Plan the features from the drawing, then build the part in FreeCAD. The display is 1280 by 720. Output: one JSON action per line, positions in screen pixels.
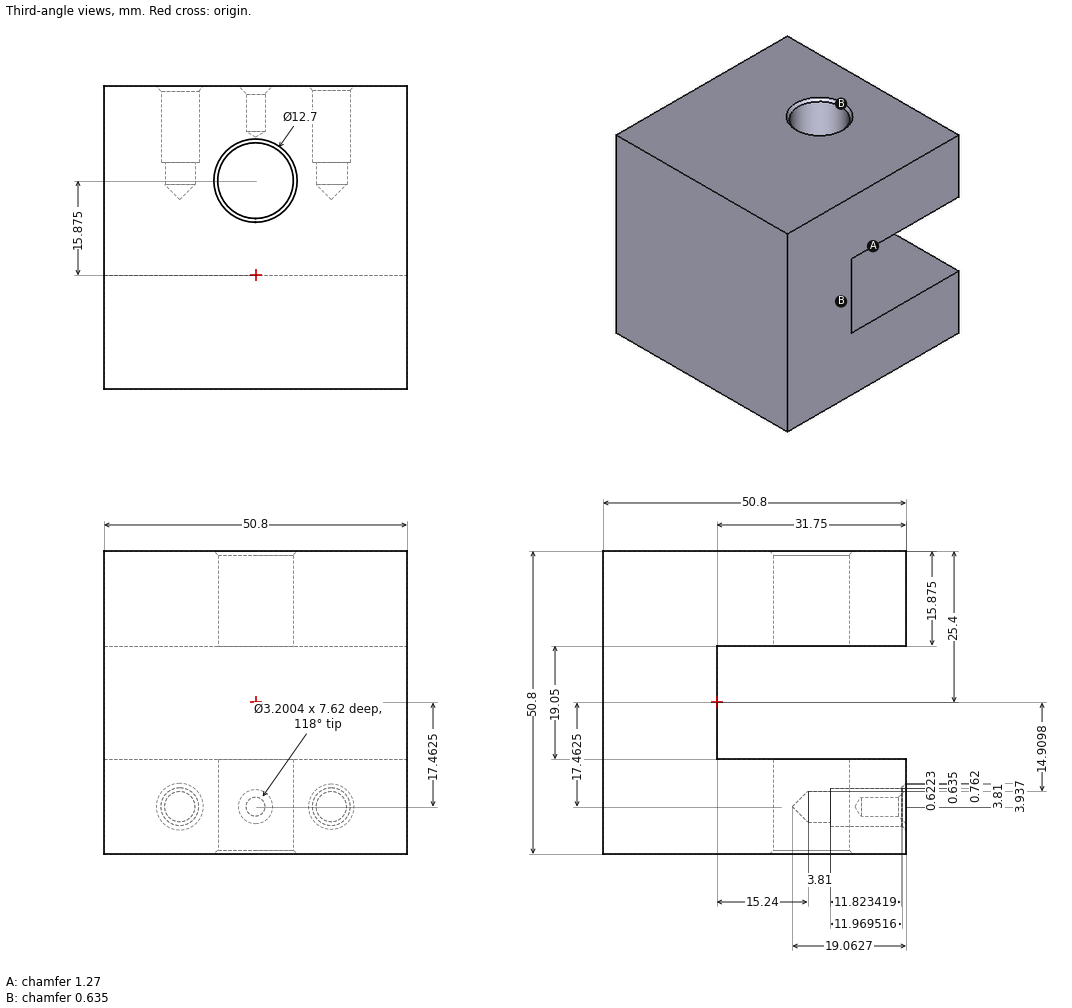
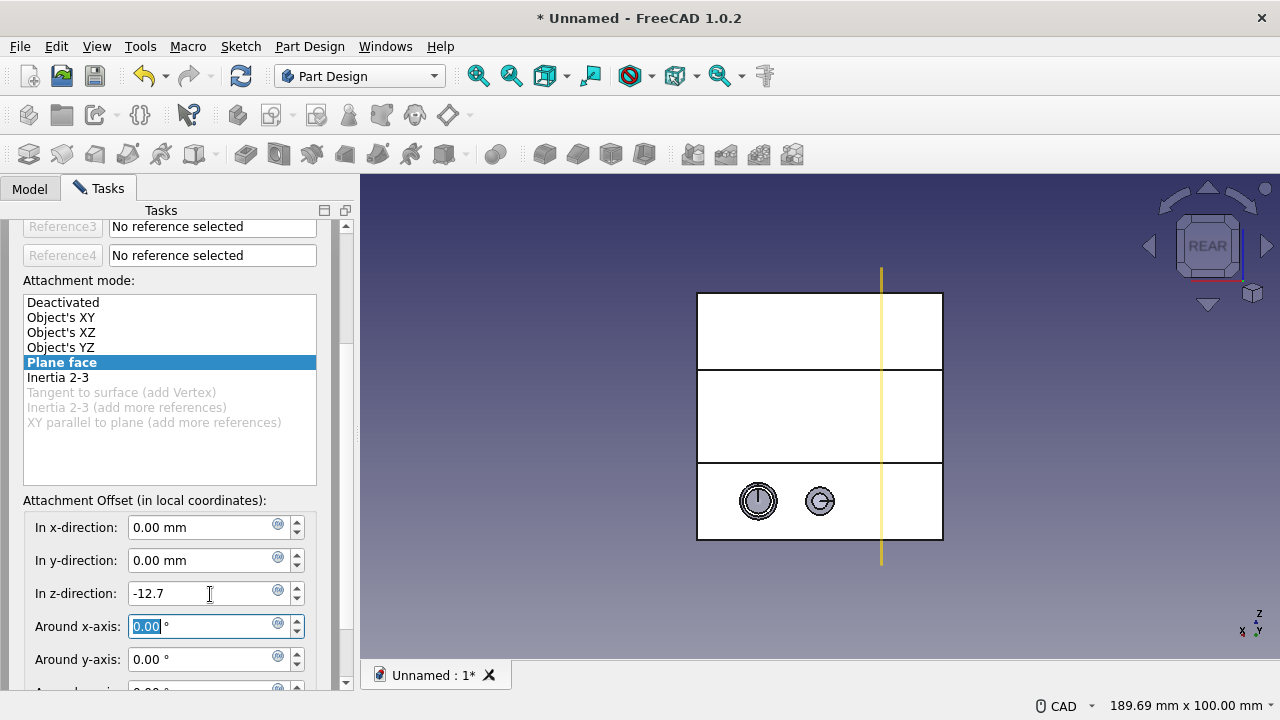
{"action": "scroll", "coordinate": [346, 455], "scroll_direction": "up", "scroll_amount": 4}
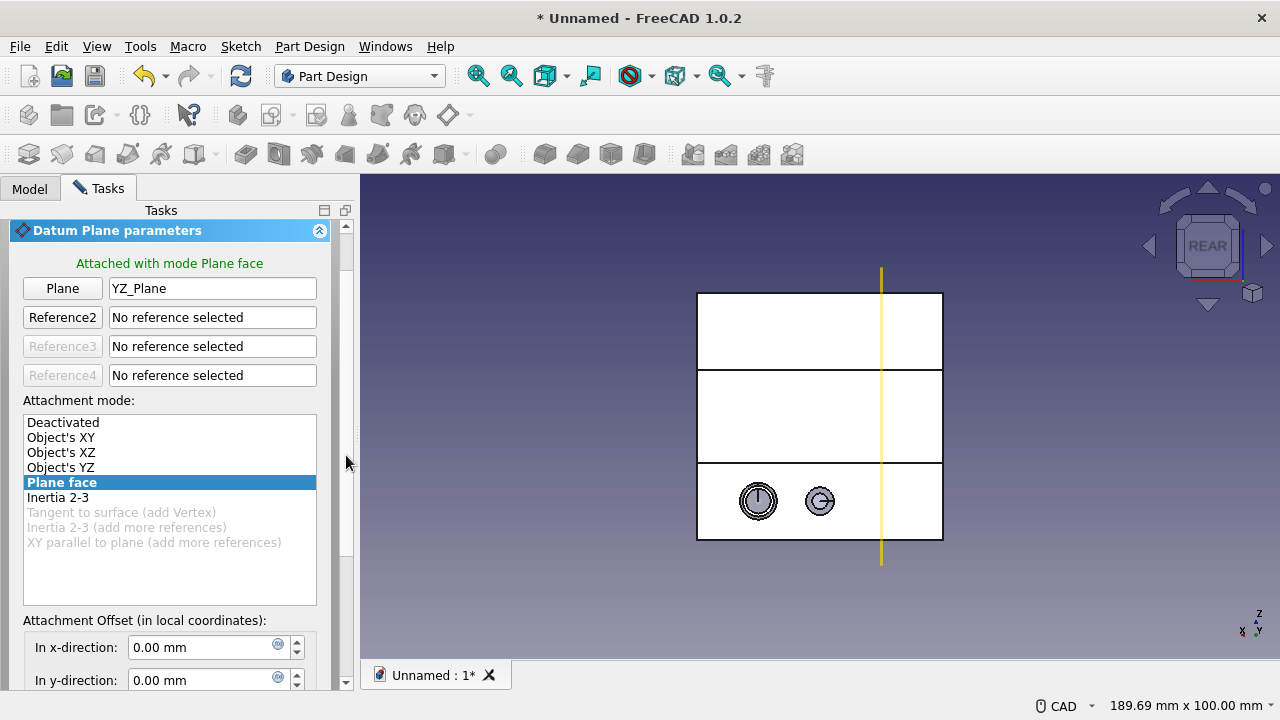
{"action": "left_click", "coordinate": [127, 249]}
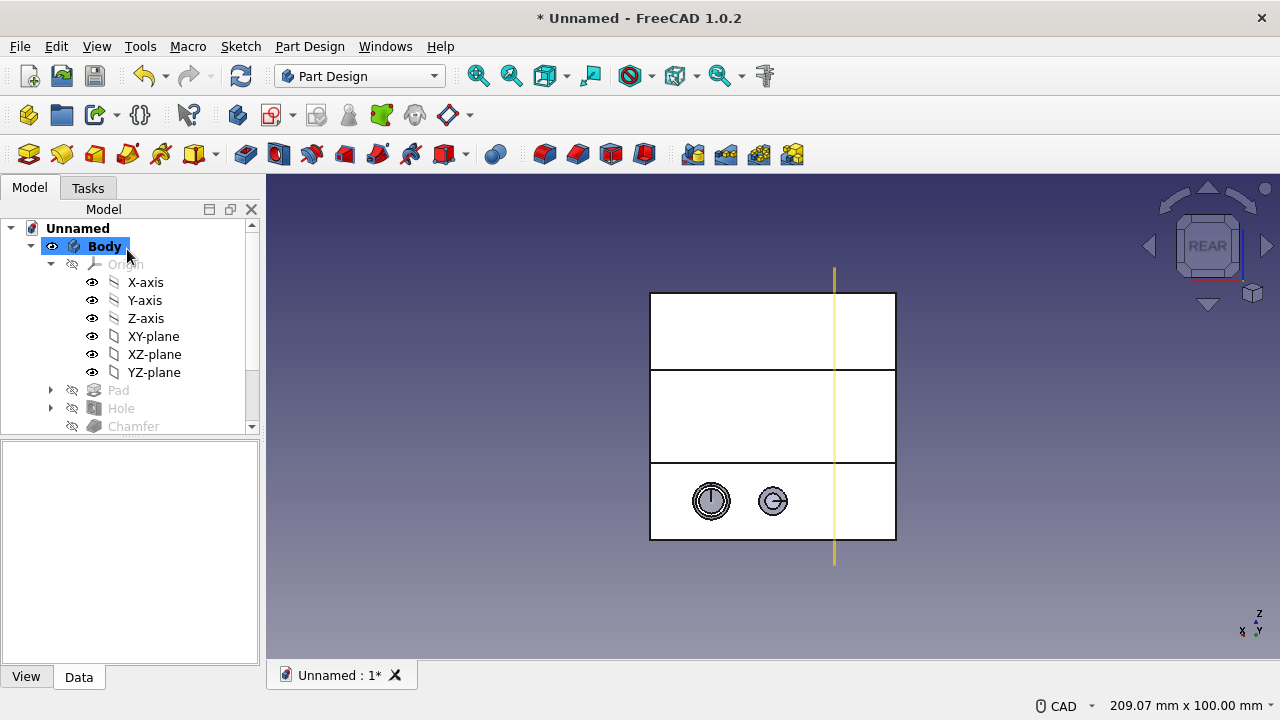
{"action": "scroll", "coordinate": [101, 332], "scroll_direction": "down", "scroll_amount": 3}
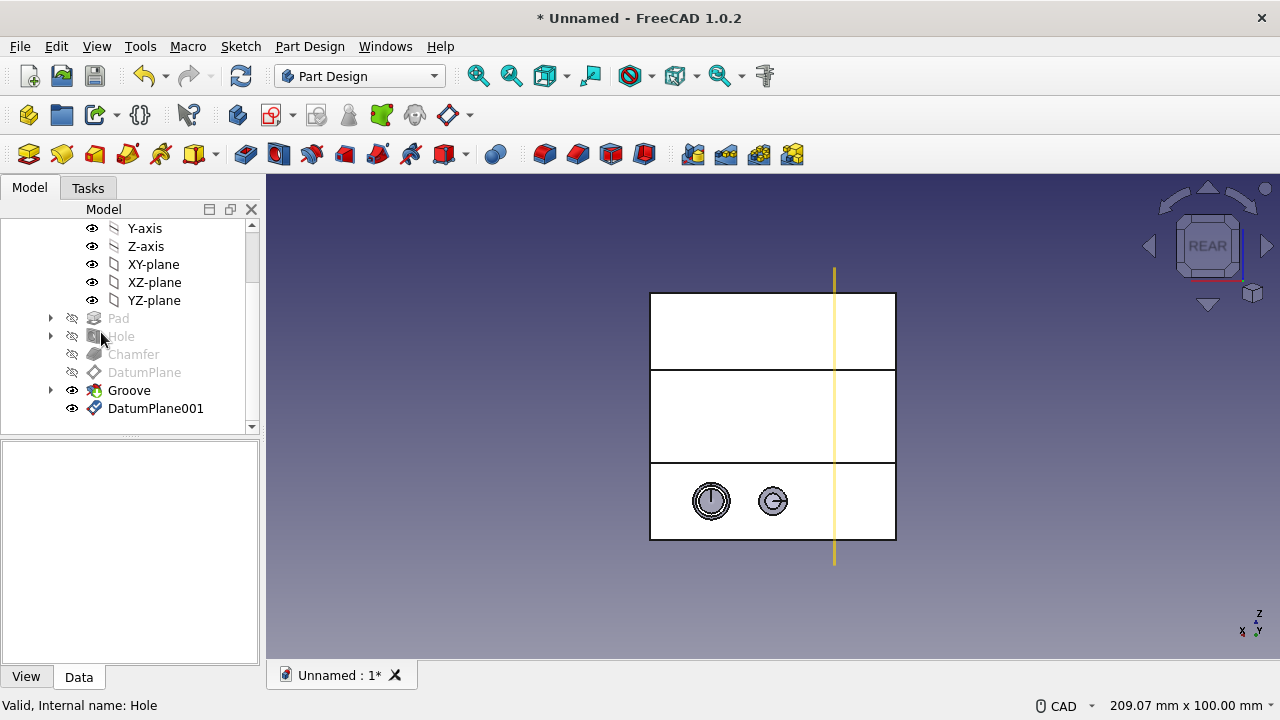
{"action": "left_click", "coordinate": [117, 408]}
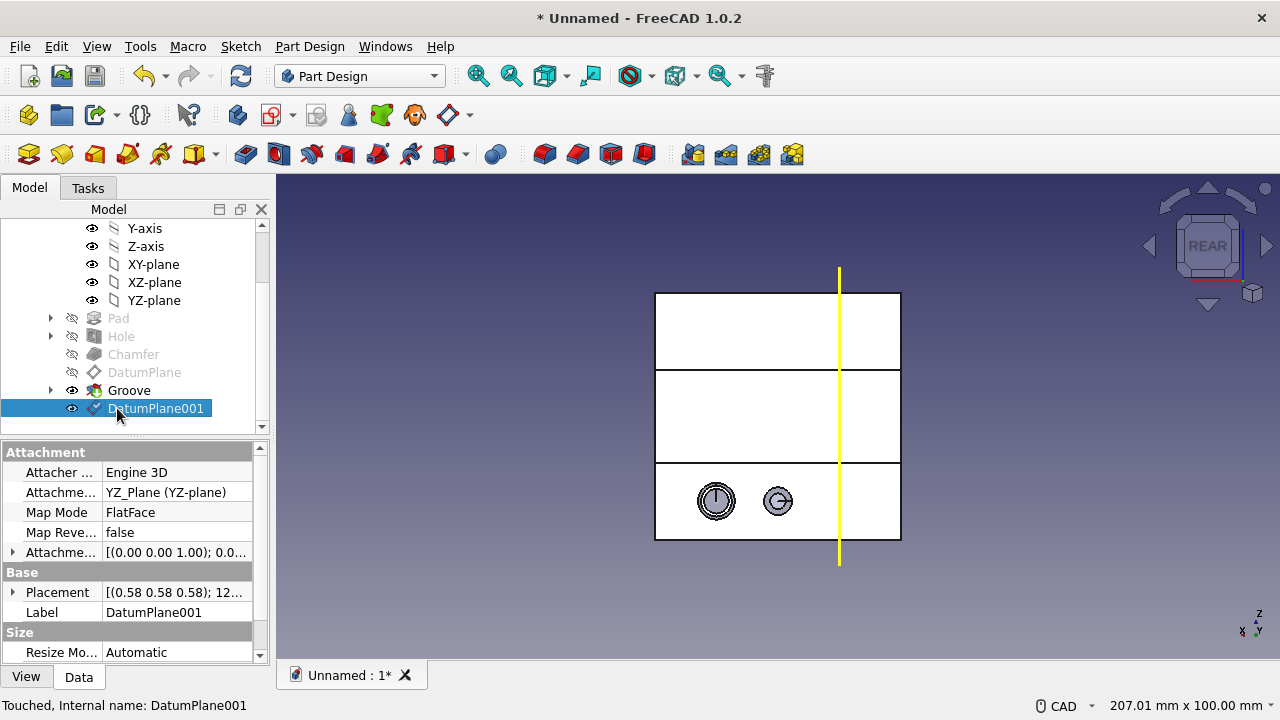
{"action": "left_click", "coordinate": [270, 116]}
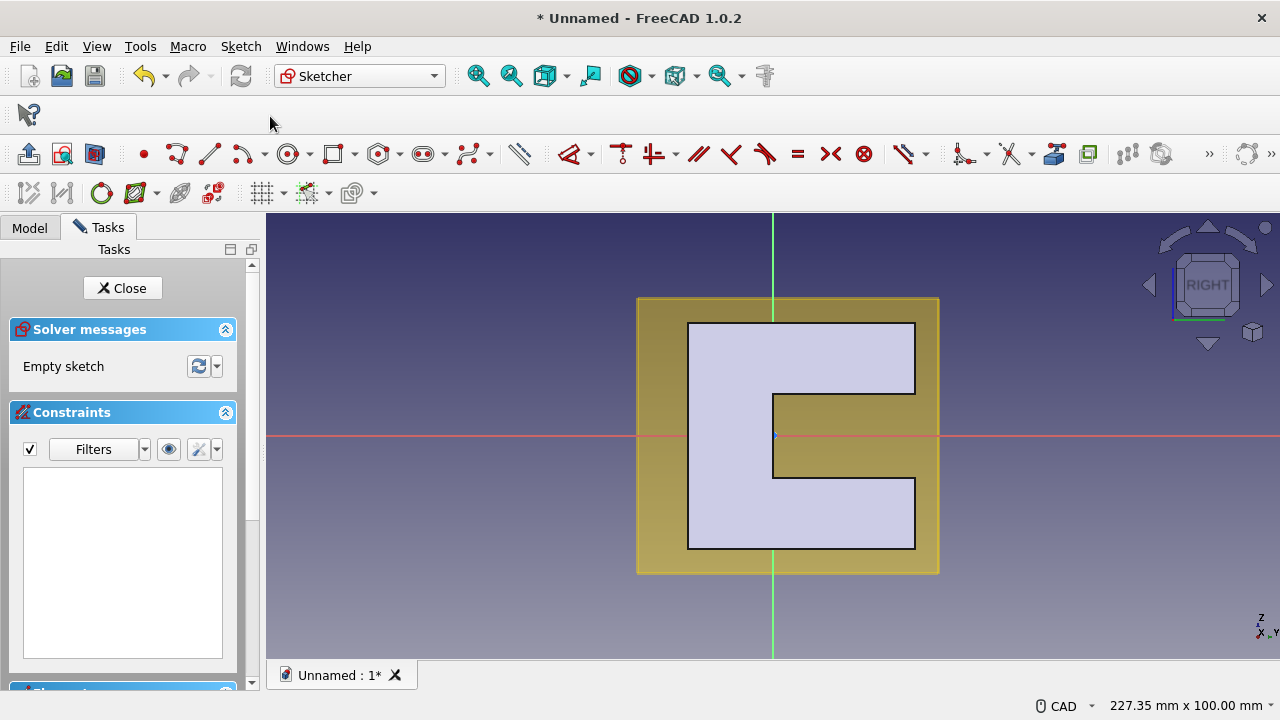
{"action": "left_click", "coordinate": [95, 154]}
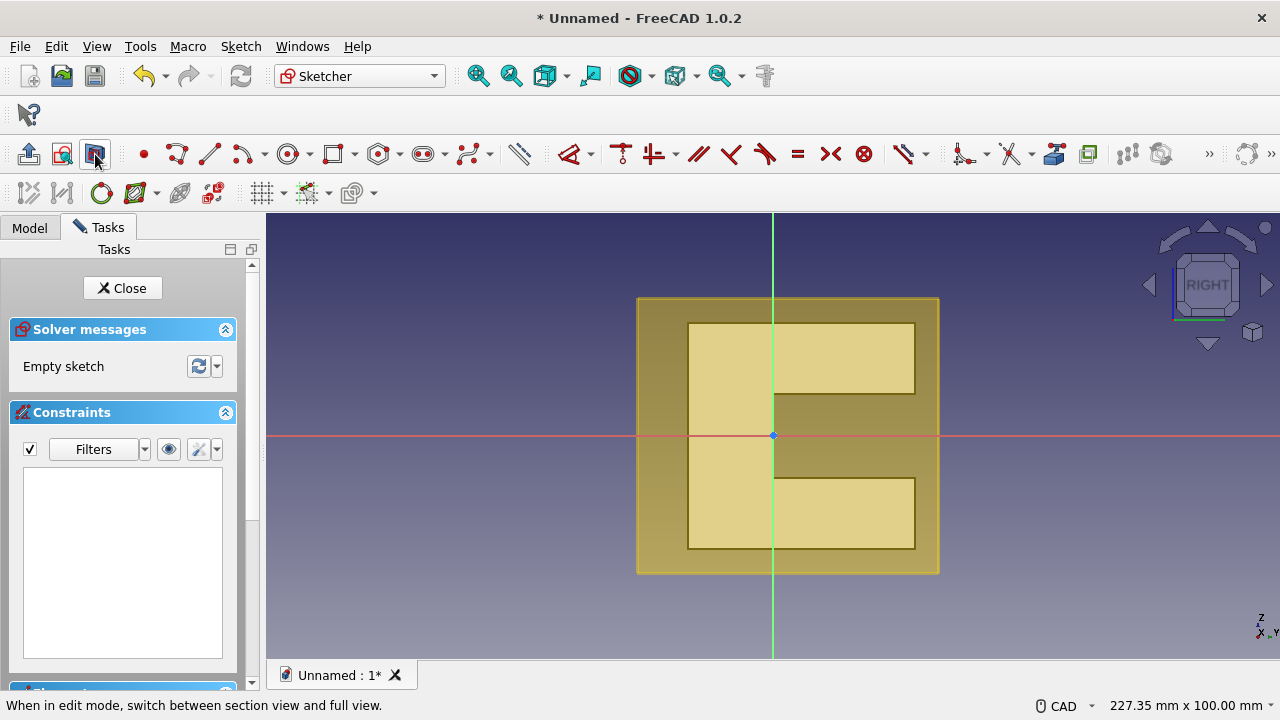
{"action": "scroll", "coordinate": [904, 492], "scroll_direction": "up", "scroll_amount": 6}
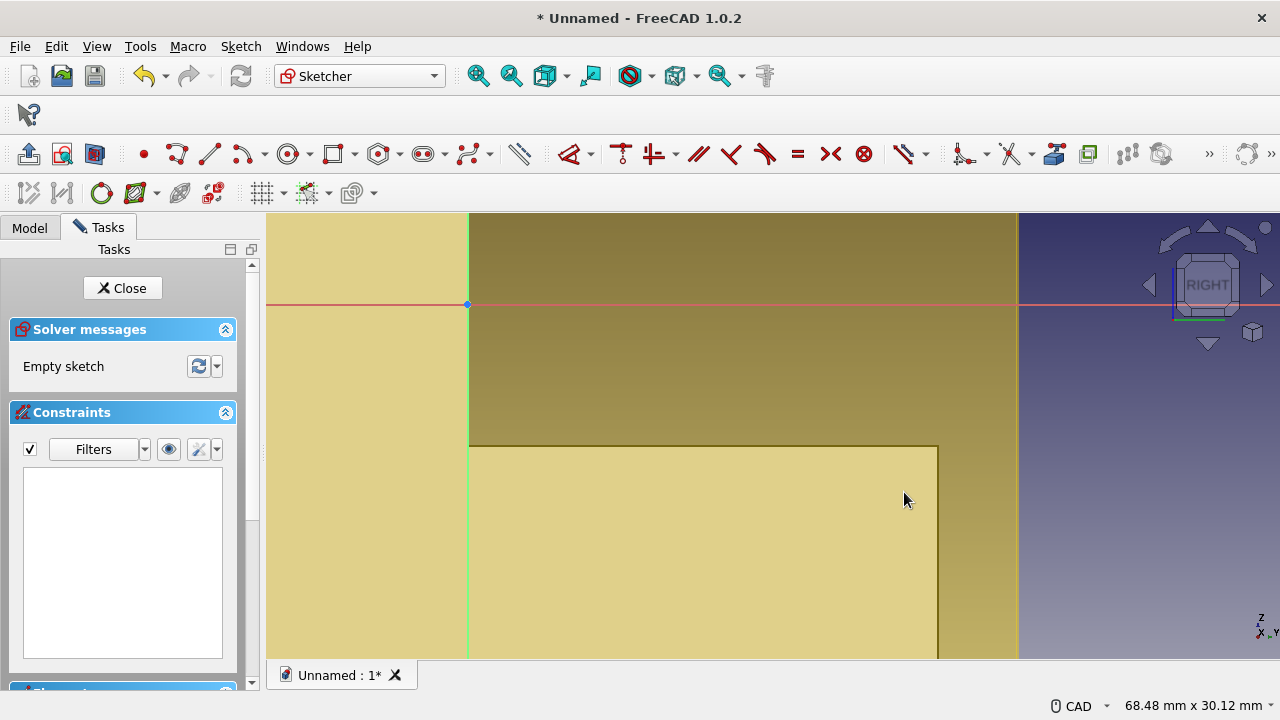
{"action": "left_click", "coordinate": [177, 154]}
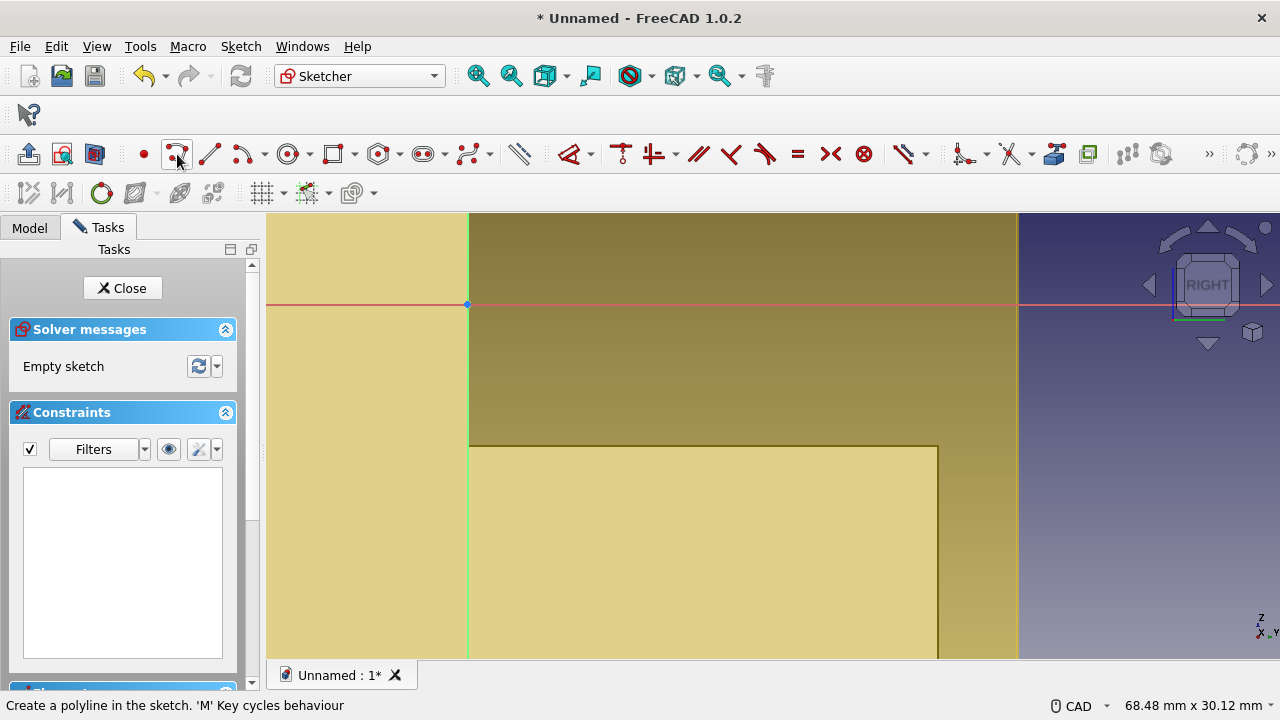
{"action": "left_click", "coordinate": [693, 525]}
{"action": "left_click", "coordinate": [655, 563]}
{"action": "left_click", "coordinate": [938, 563]}
{"action": "left_click", "coordinate": [938, 505]}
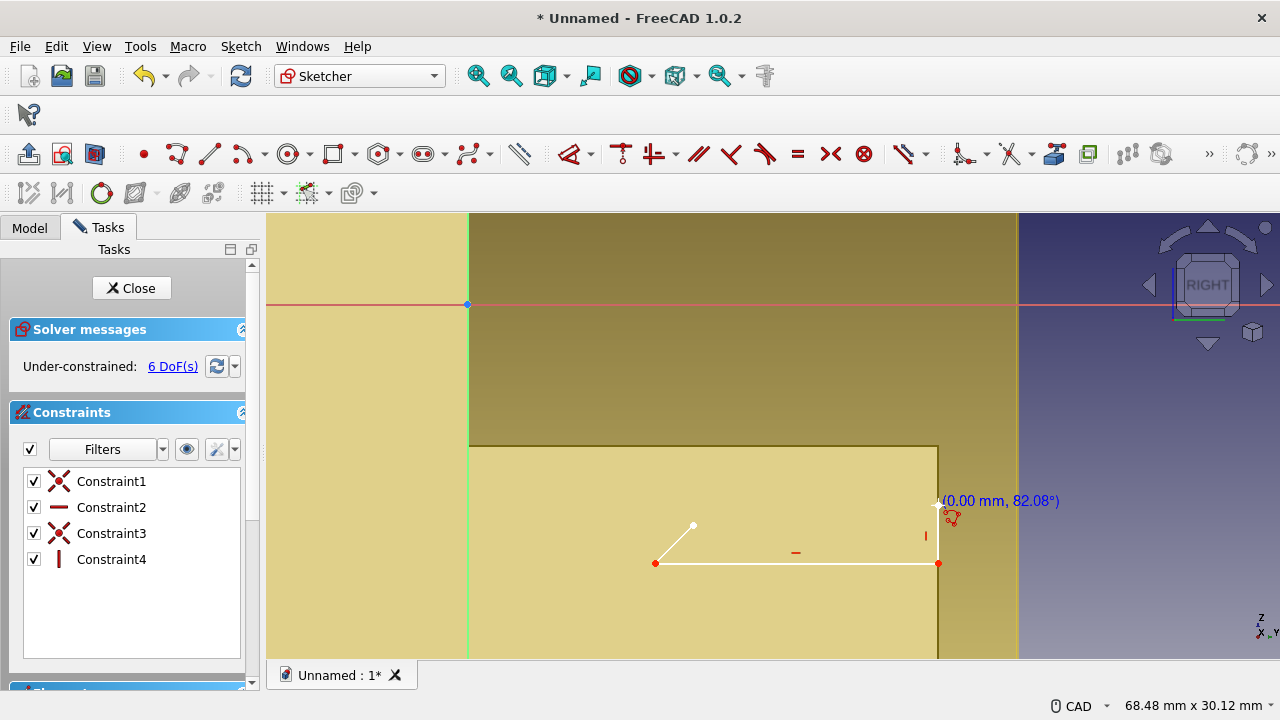
{"action": "scroll", "coordinate": [925, 516], "scroll_direction": "up", "scroll_amount": 2}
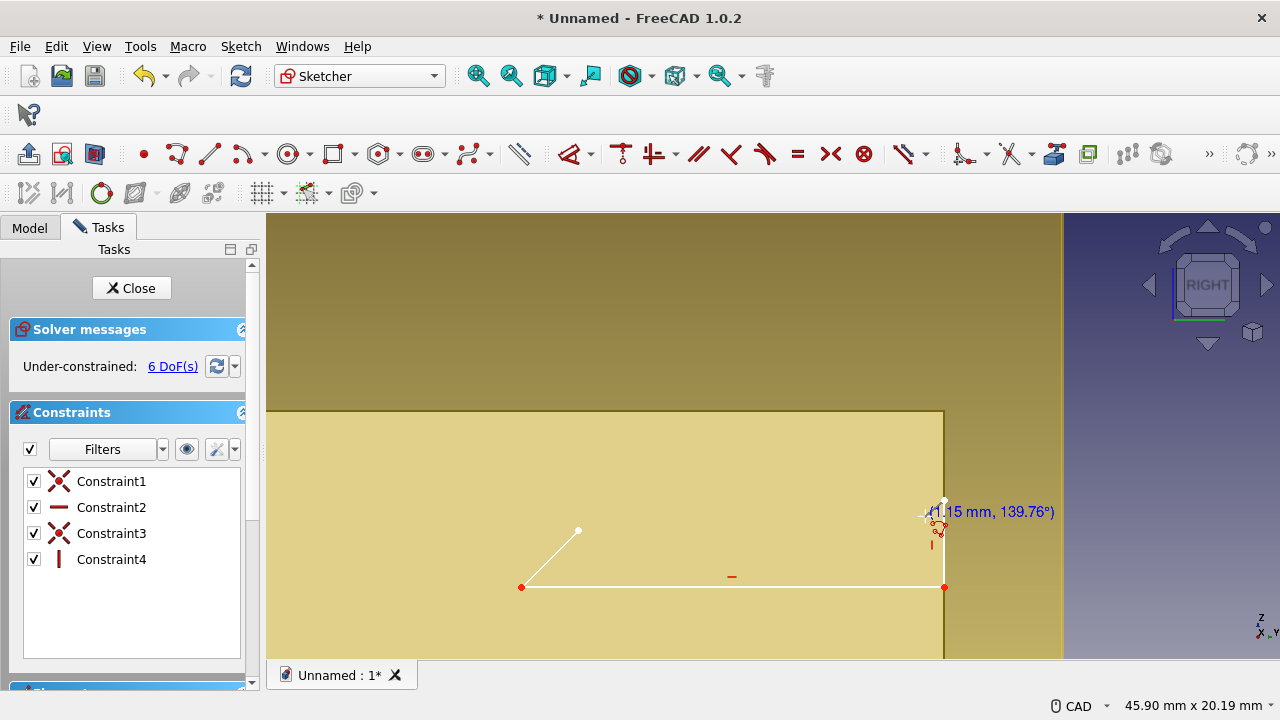
{"action": "left_click", "coordinate": [924, 516]}
{"action": "left_click", "coordinate": [663, 516]}
{"action": "left_click", "coordinate": [663, 530]}
{"action": "left_click", "coordinate": [579, 531]}